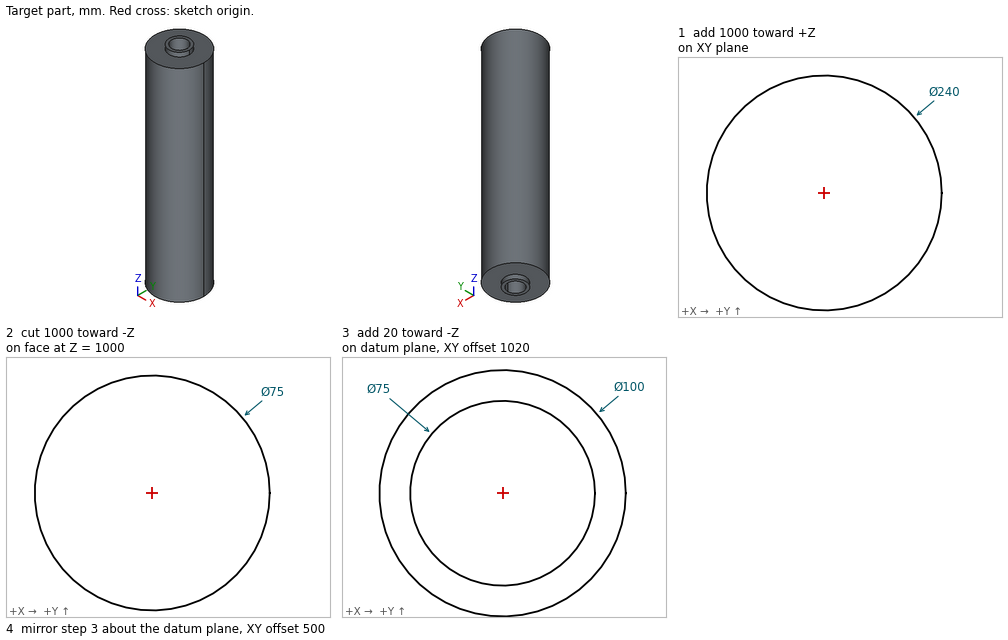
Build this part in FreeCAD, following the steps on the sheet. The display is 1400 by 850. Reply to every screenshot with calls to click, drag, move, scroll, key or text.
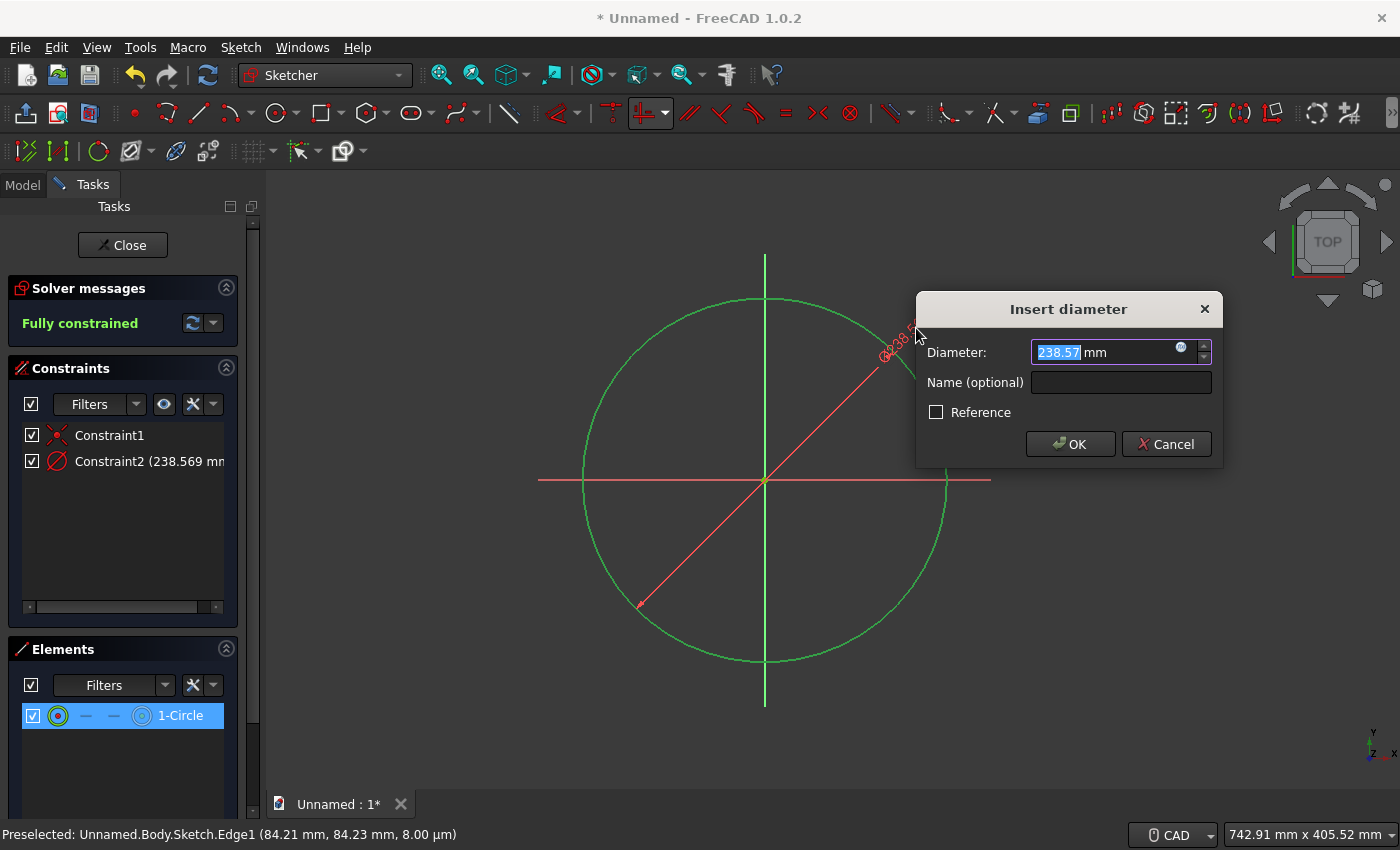
text(240)
key(Return)
key(Escape)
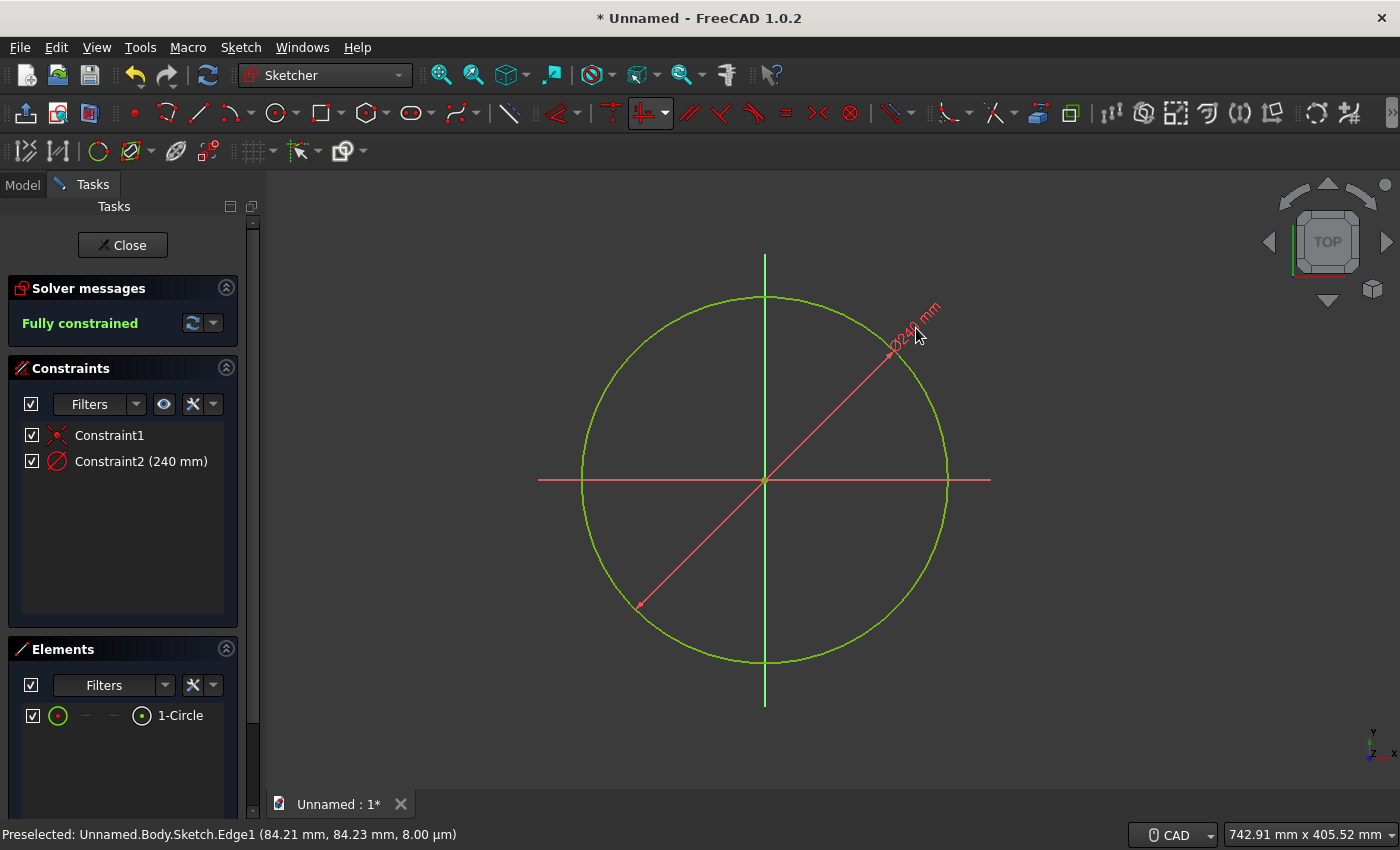
click(123, 245)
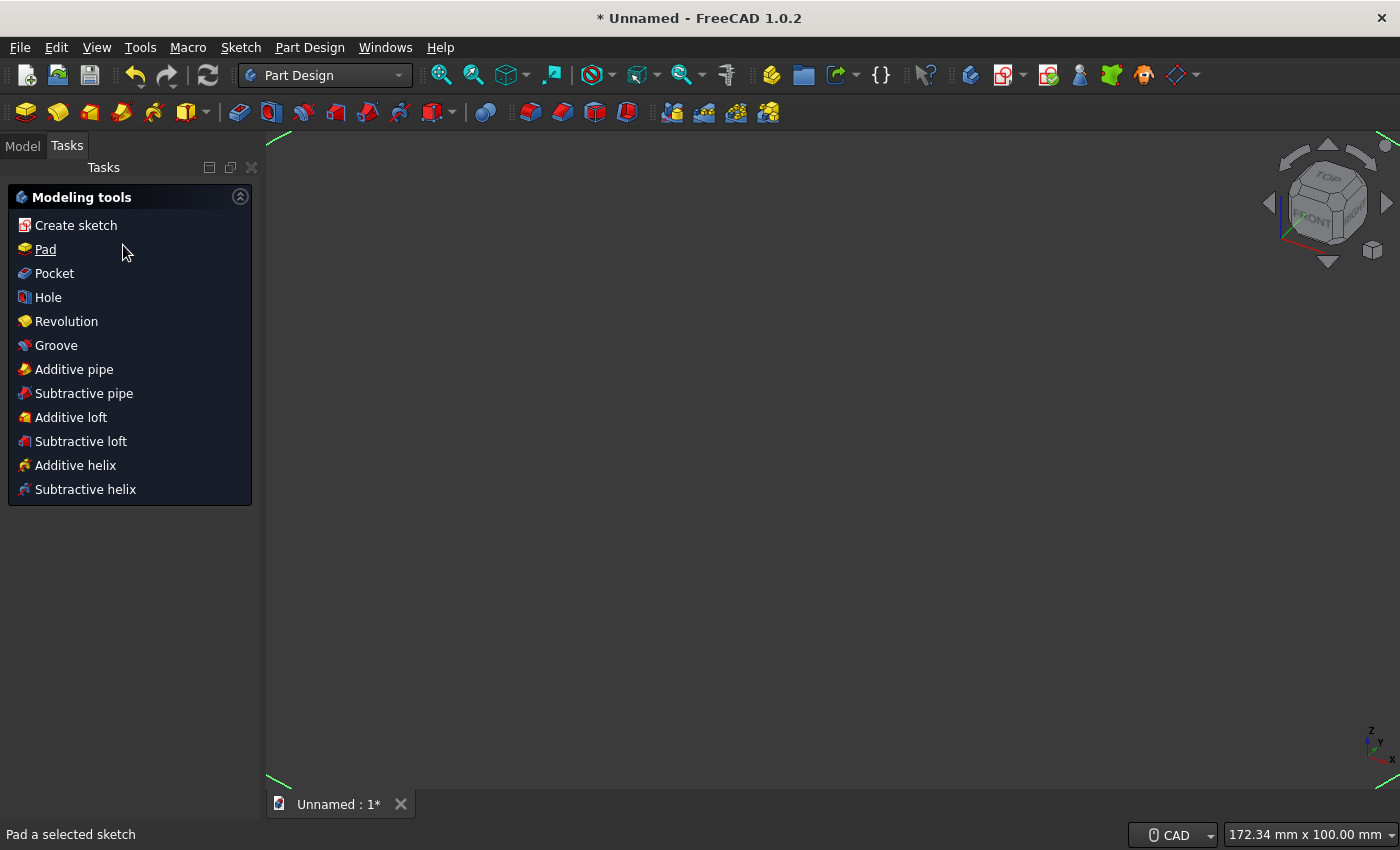
click(26, 112)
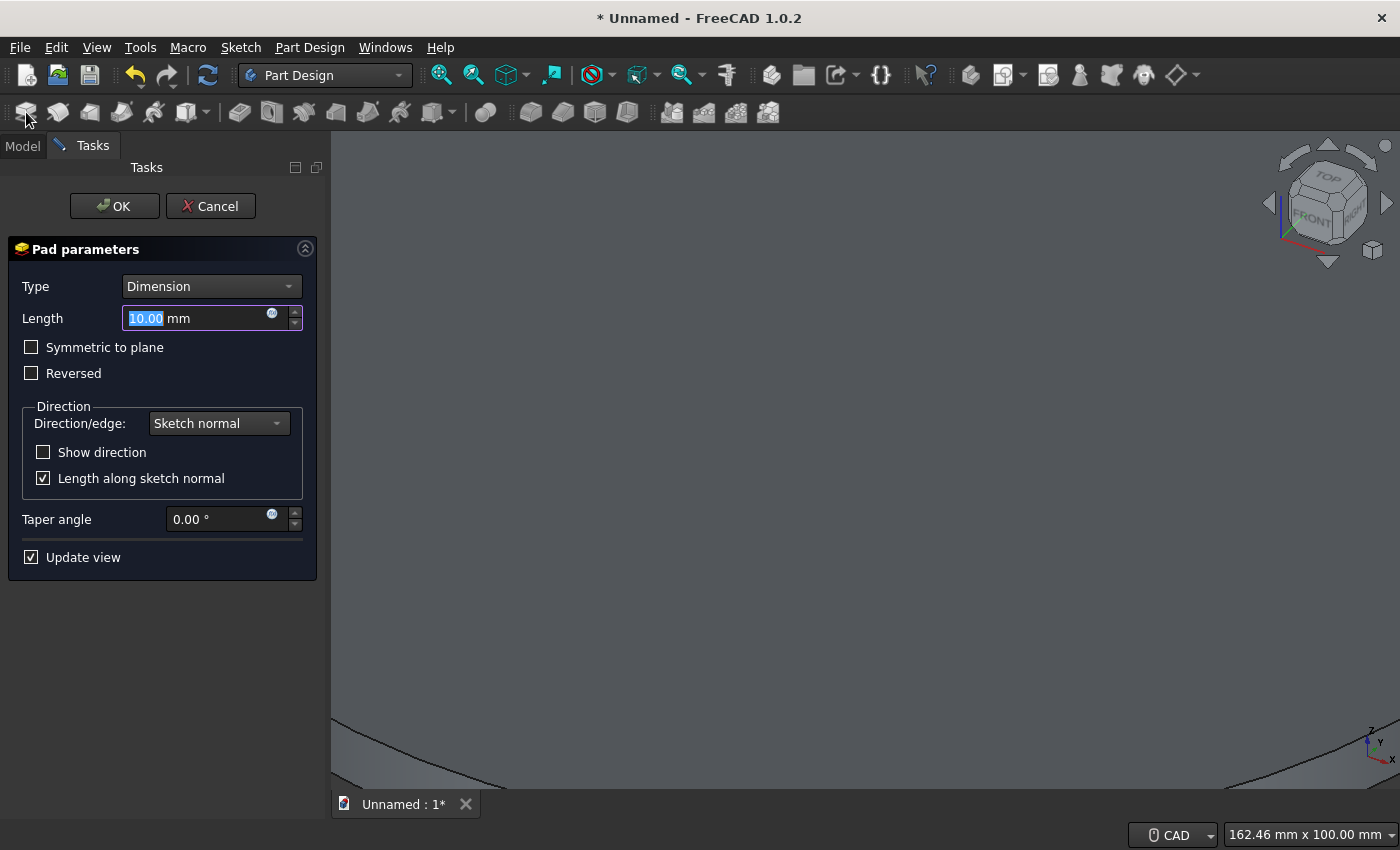
text(1000)
key(Tab)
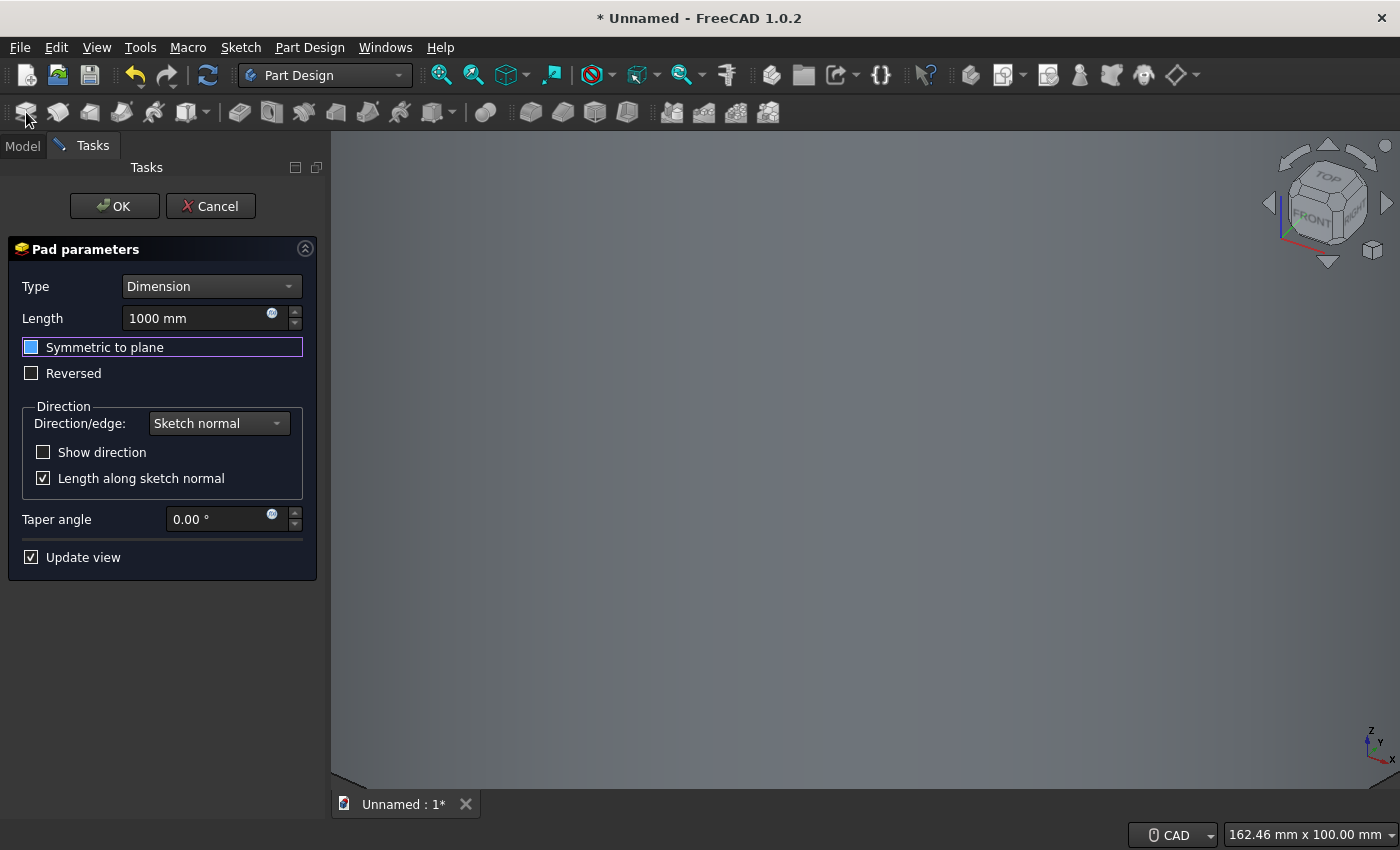
click(115, 206)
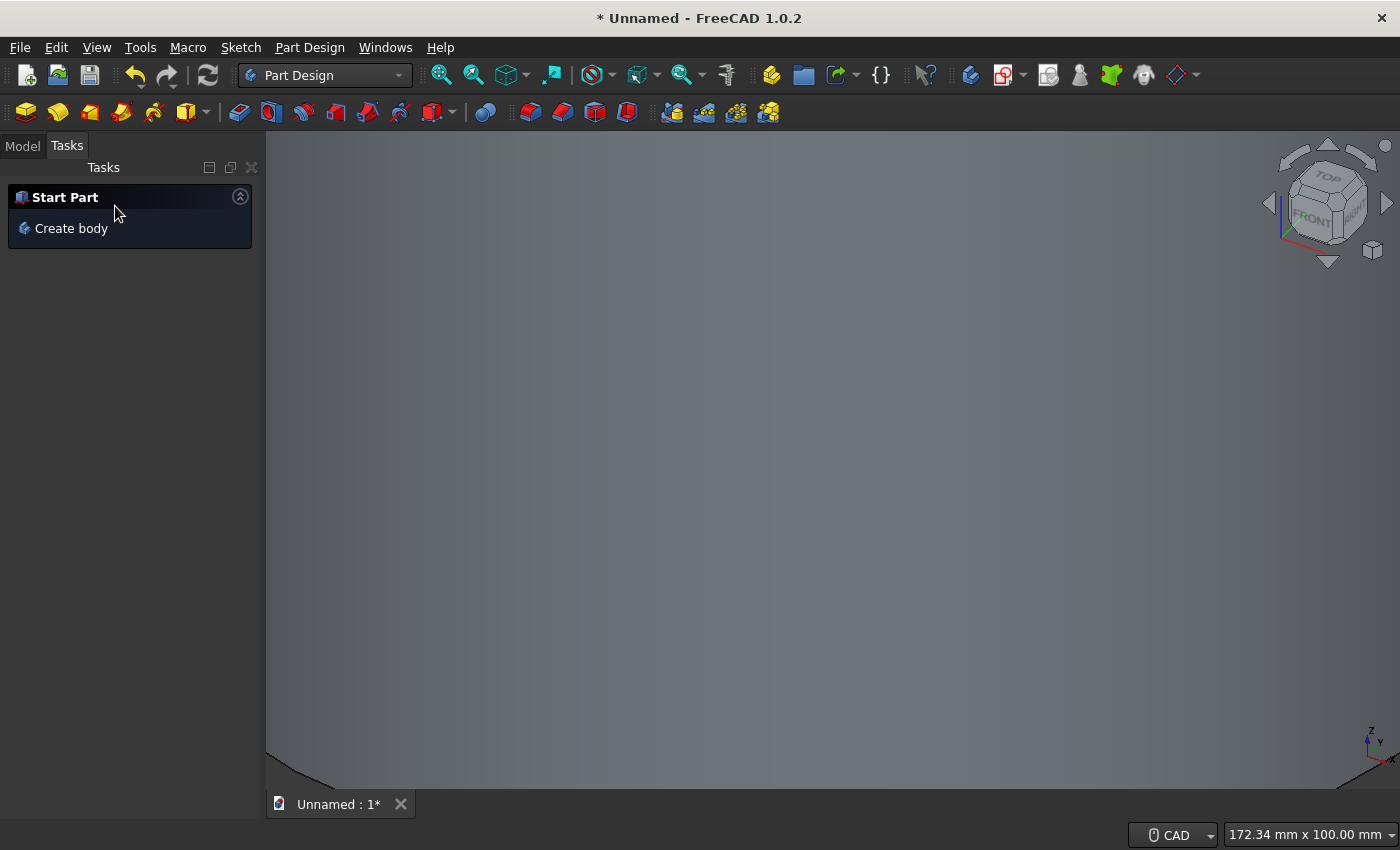
key(v)
key(f)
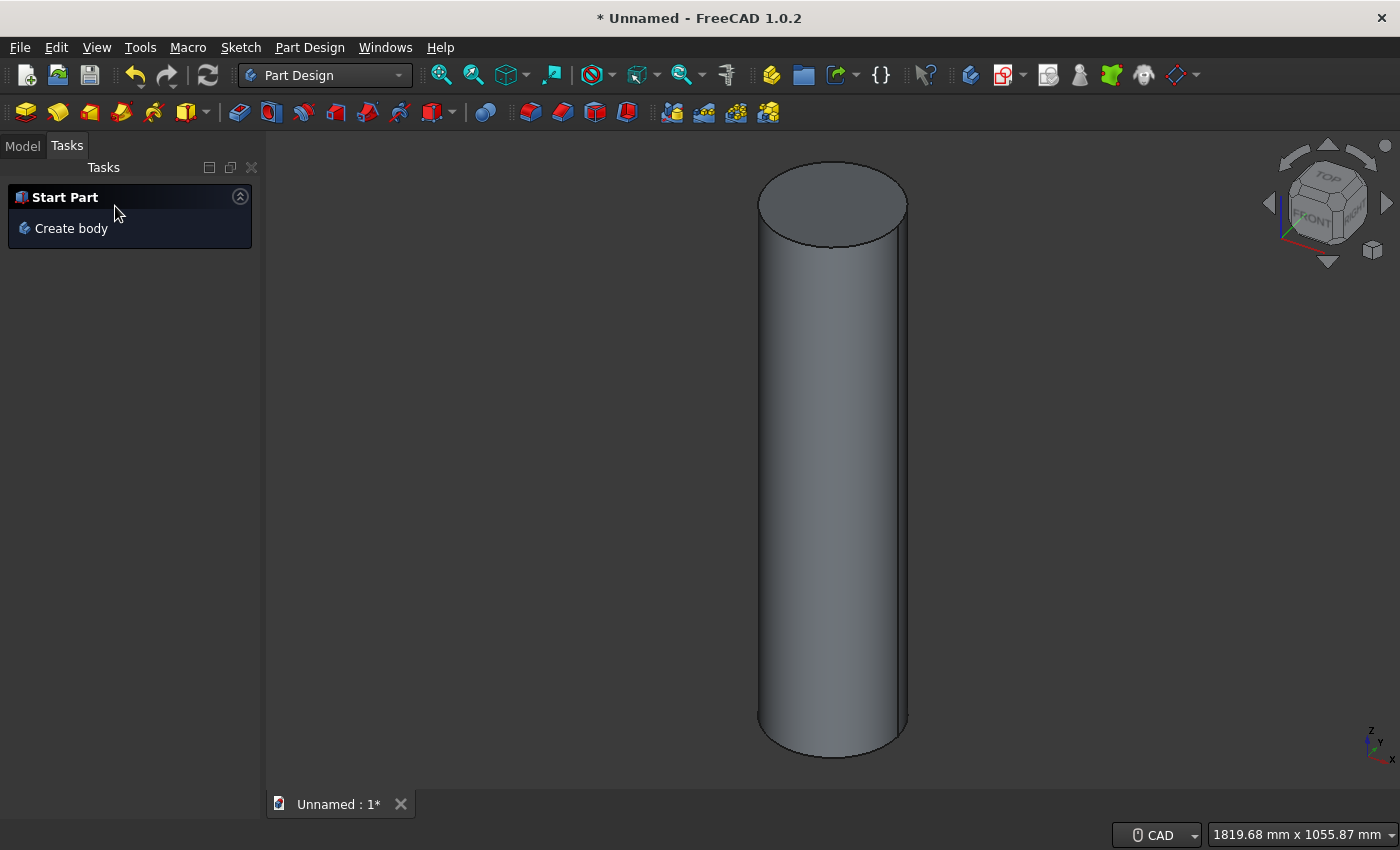
click(833, 204)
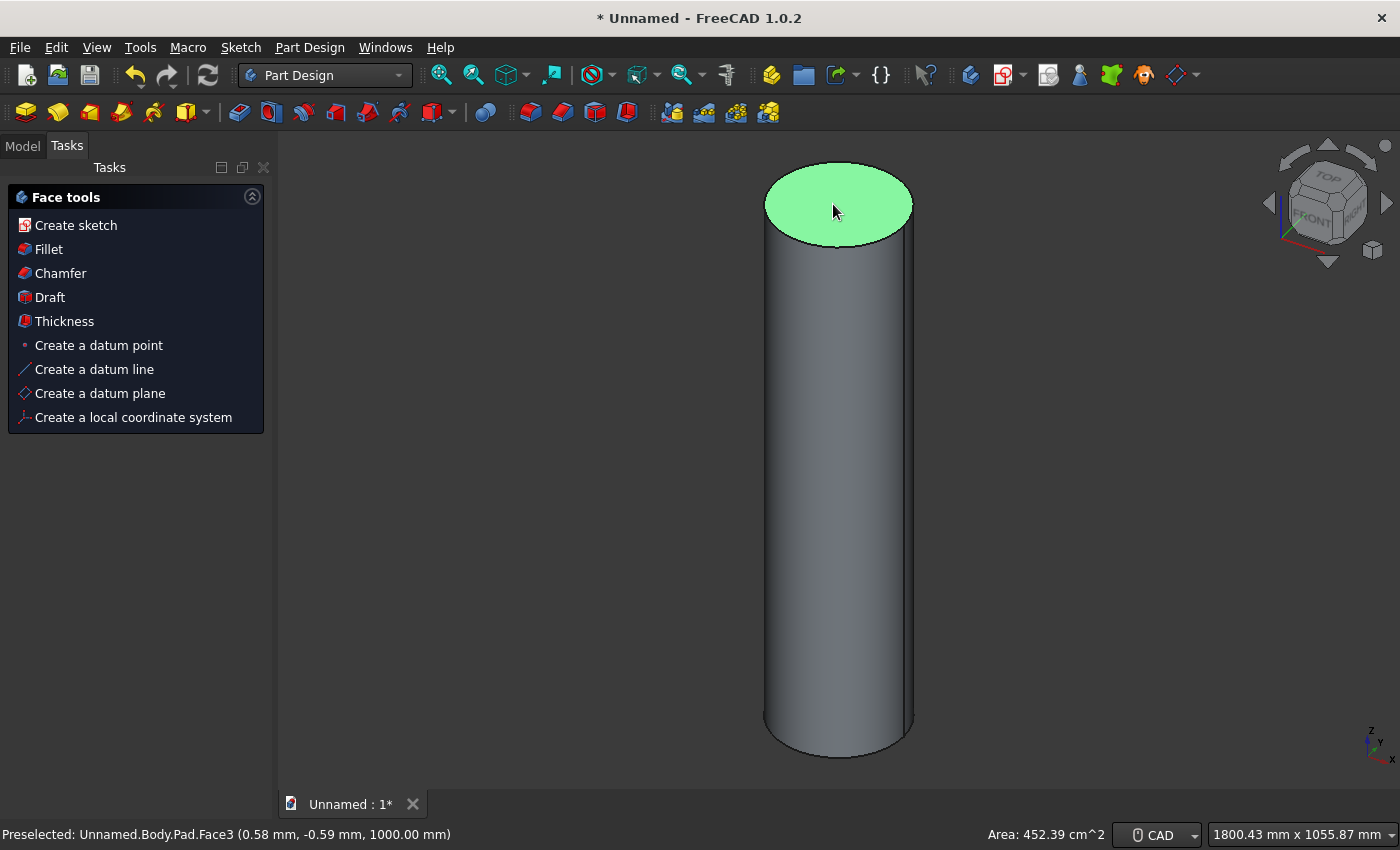
click(1004, 76)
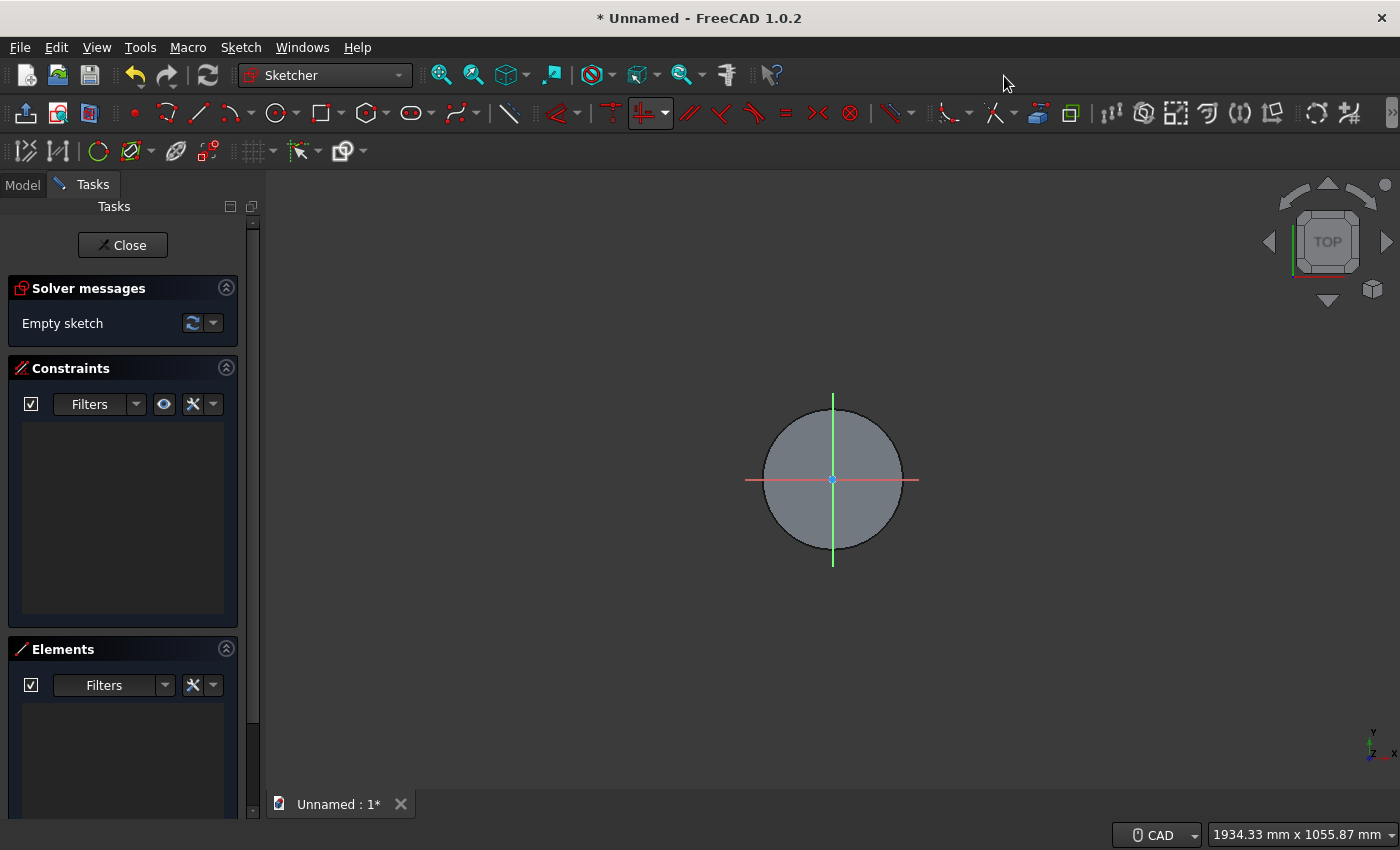
scroll(841, 479, up, 11)